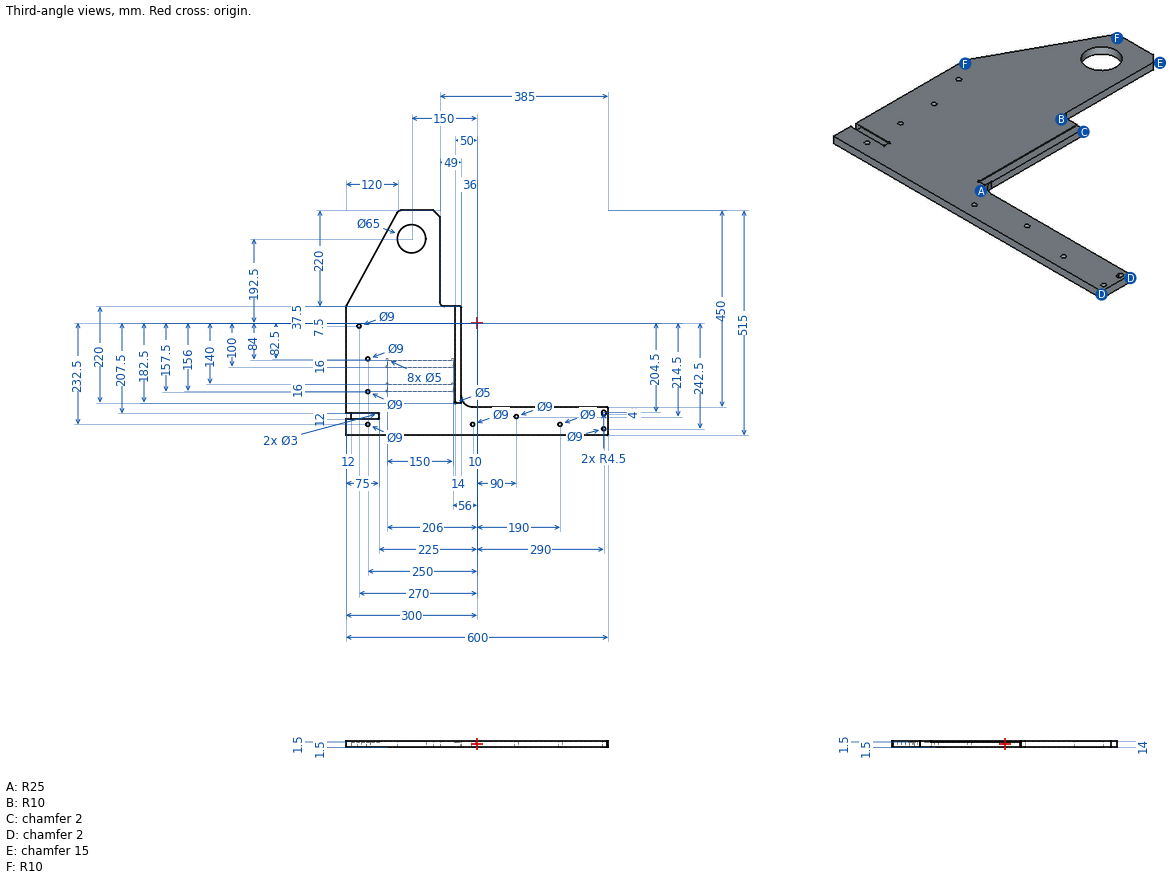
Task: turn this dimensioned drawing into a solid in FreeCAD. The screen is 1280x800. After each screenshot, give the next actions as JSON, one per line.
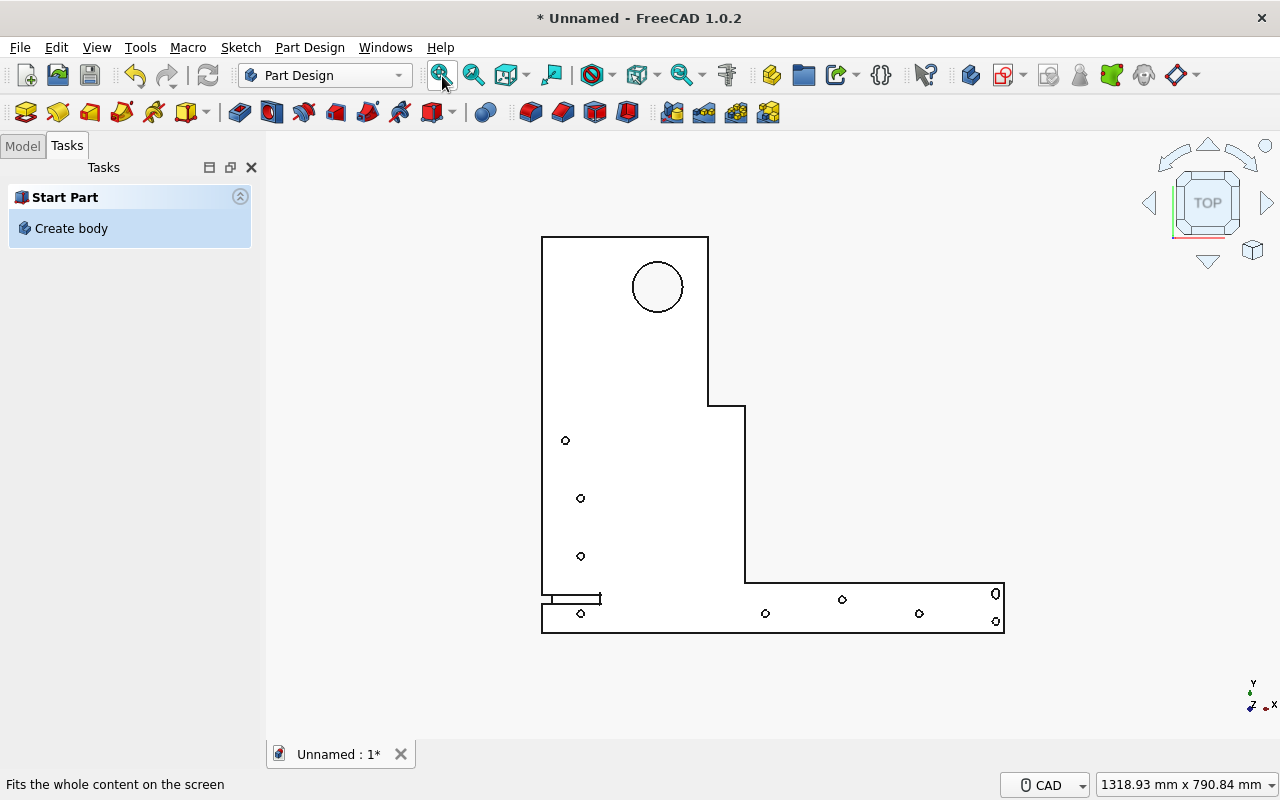
{"action": "key", "text": "1"}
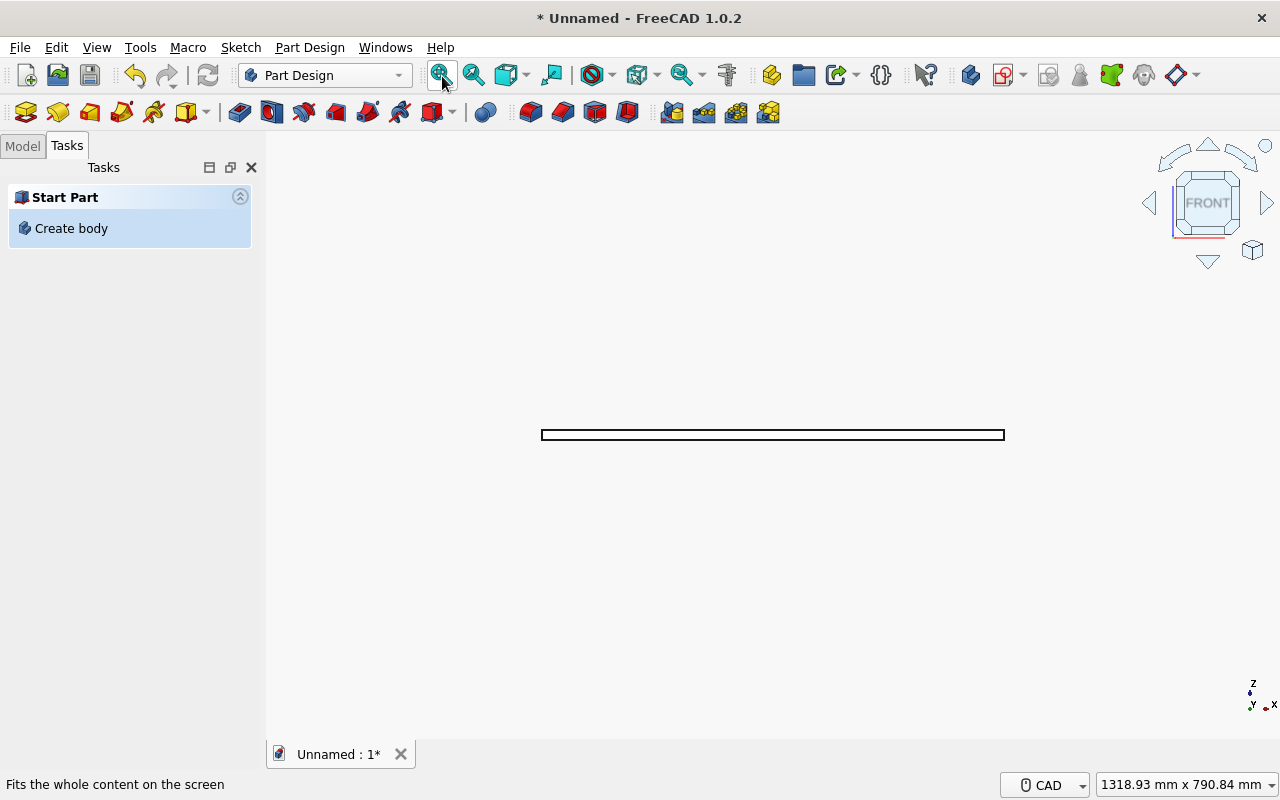
{"action": "scroll", "coordinate": [745, 434], "scroll_direction": "up", "scroll_amount": 7}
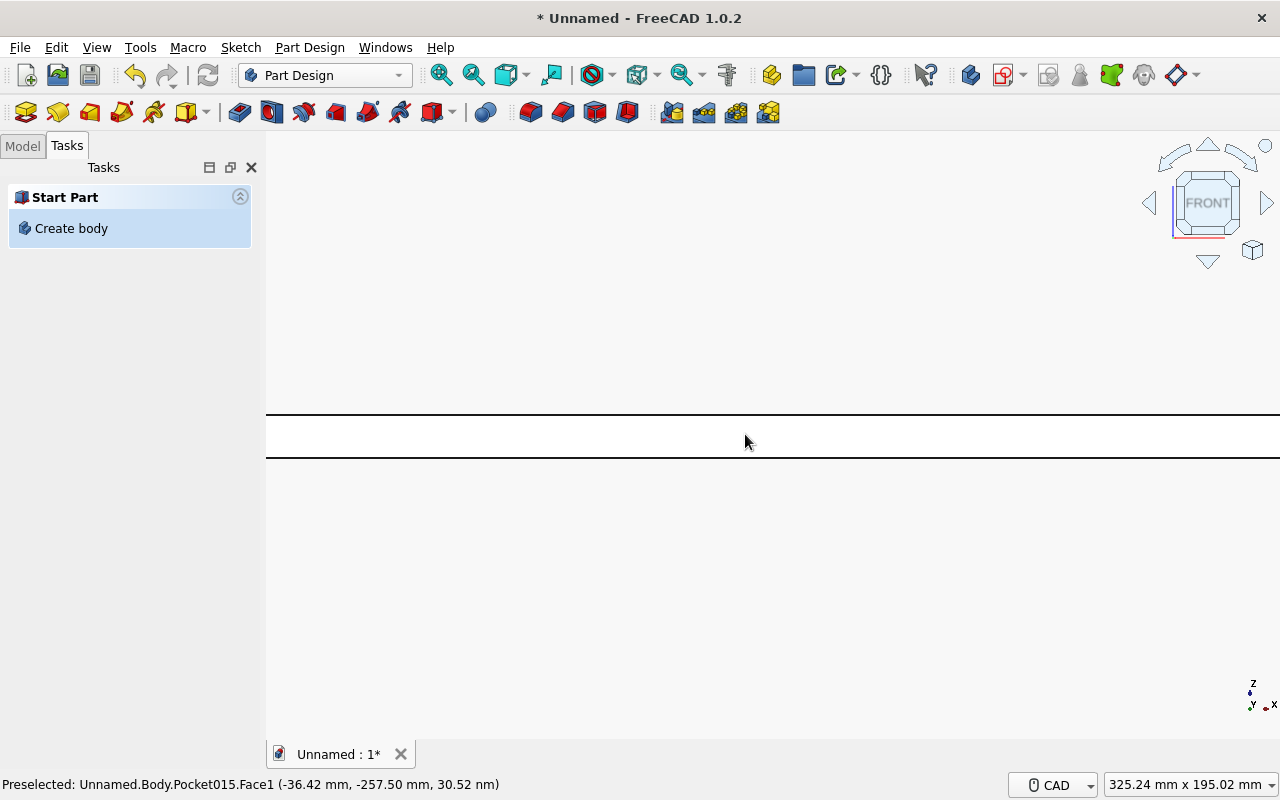
{"action": "left_click", "coordinate": [442, 76]}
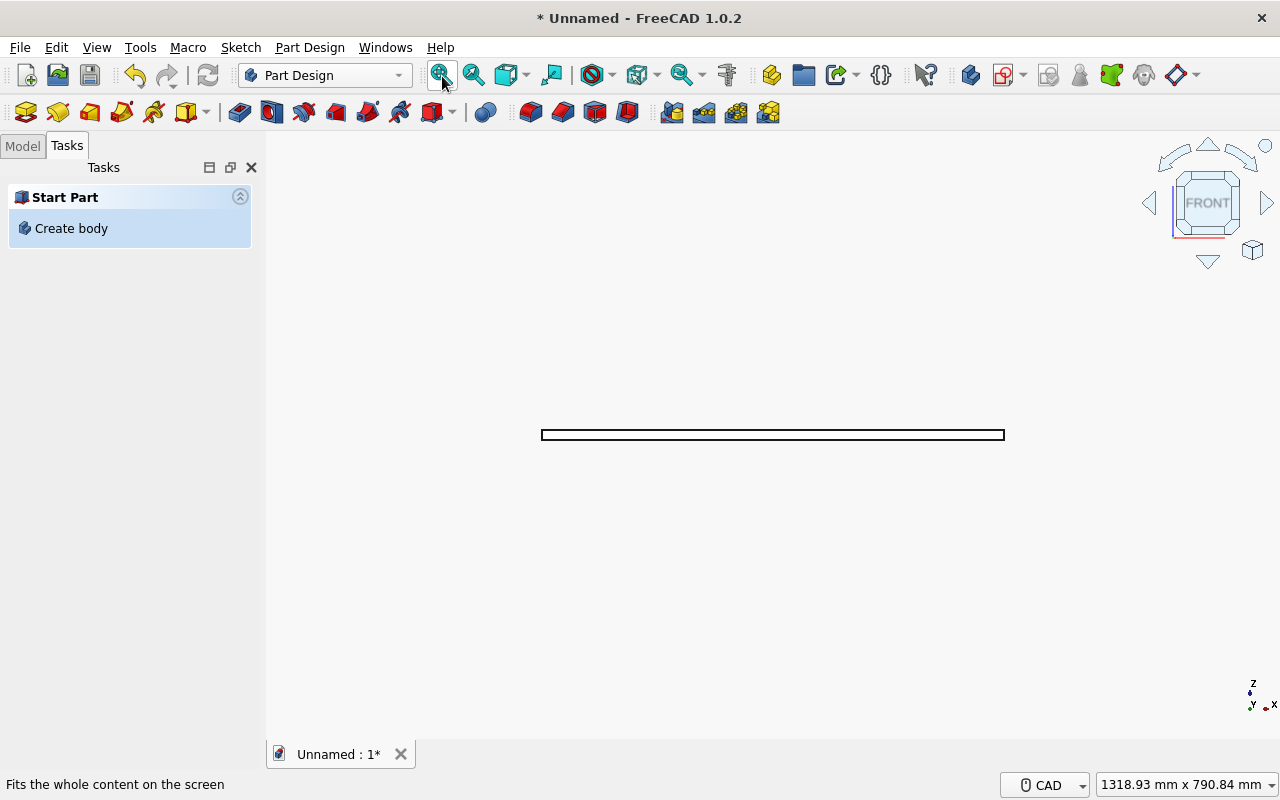
{"action": "key", "text": "3"}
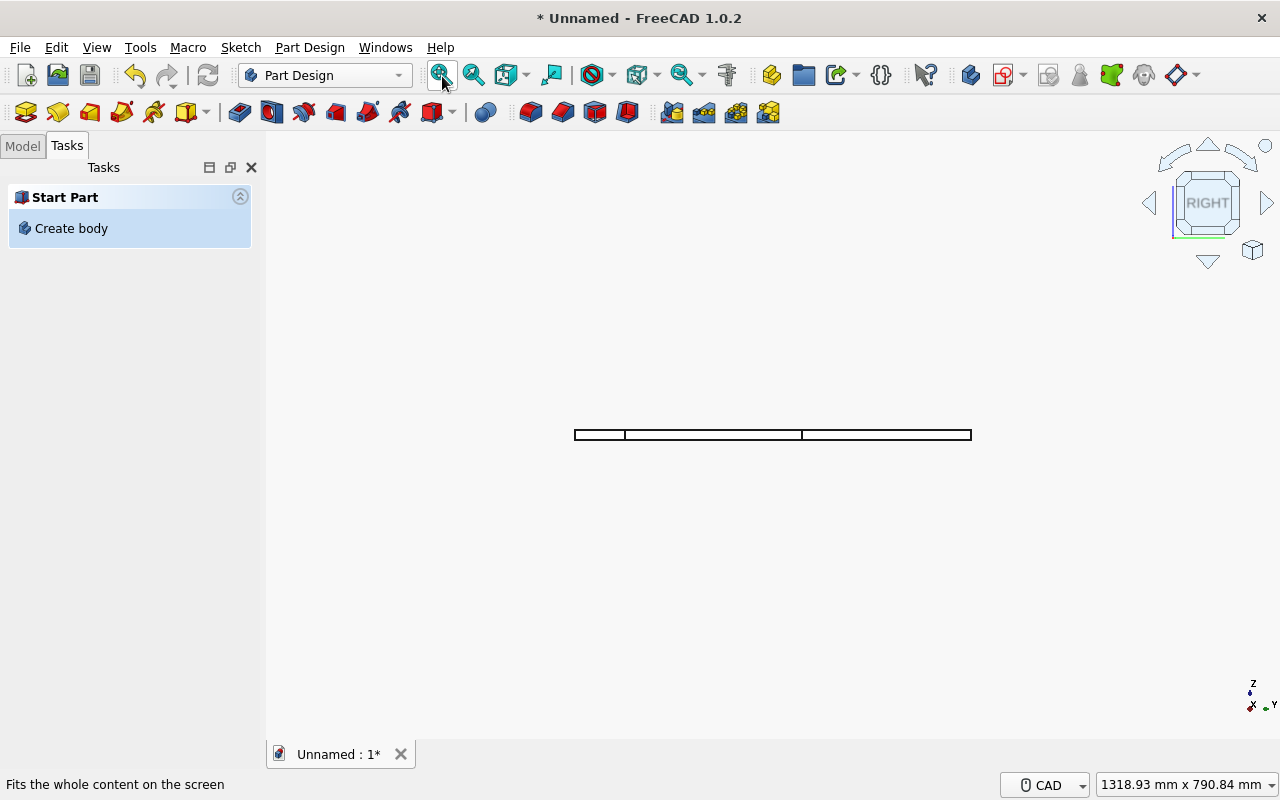
{"action": "left_click", "coordinate": [442, 76]}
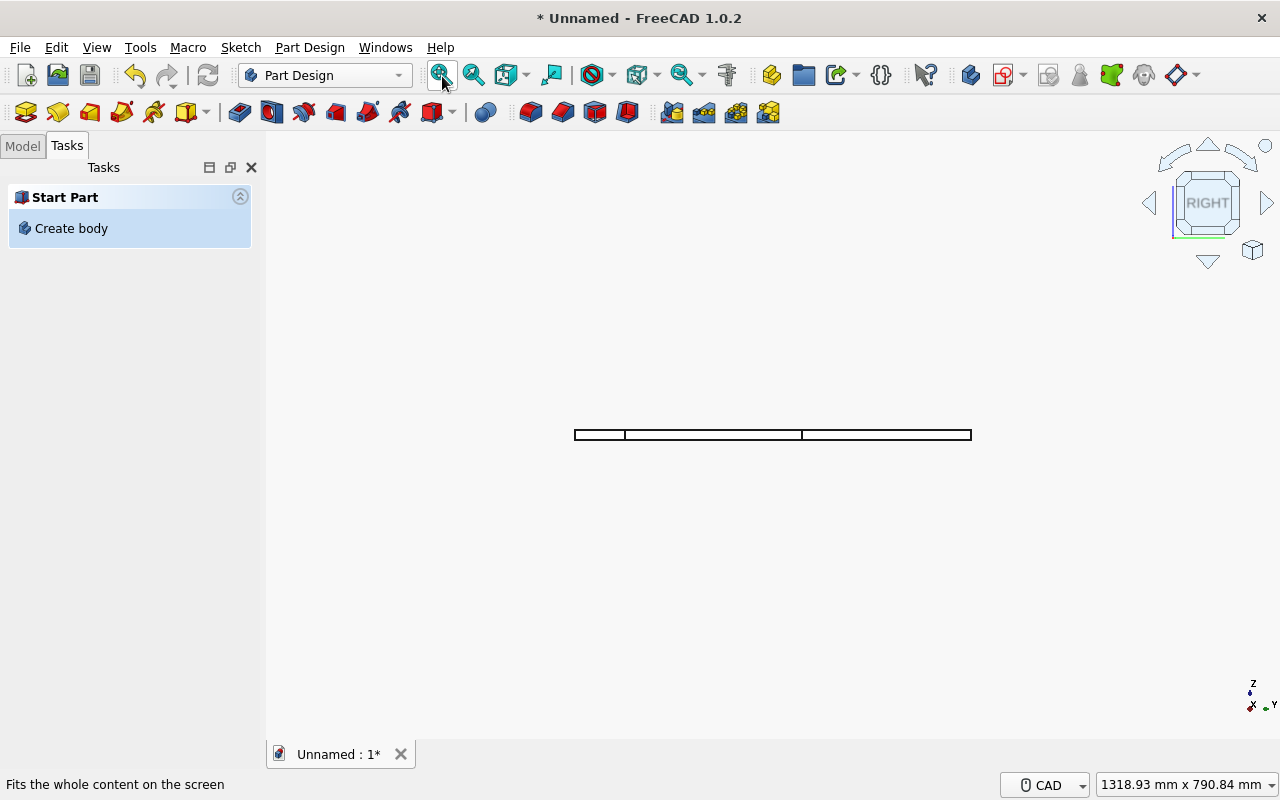
{"action": "scroll", "coordinate": [625, 434], "scroll_direction": "up", "scroll_amount": 7}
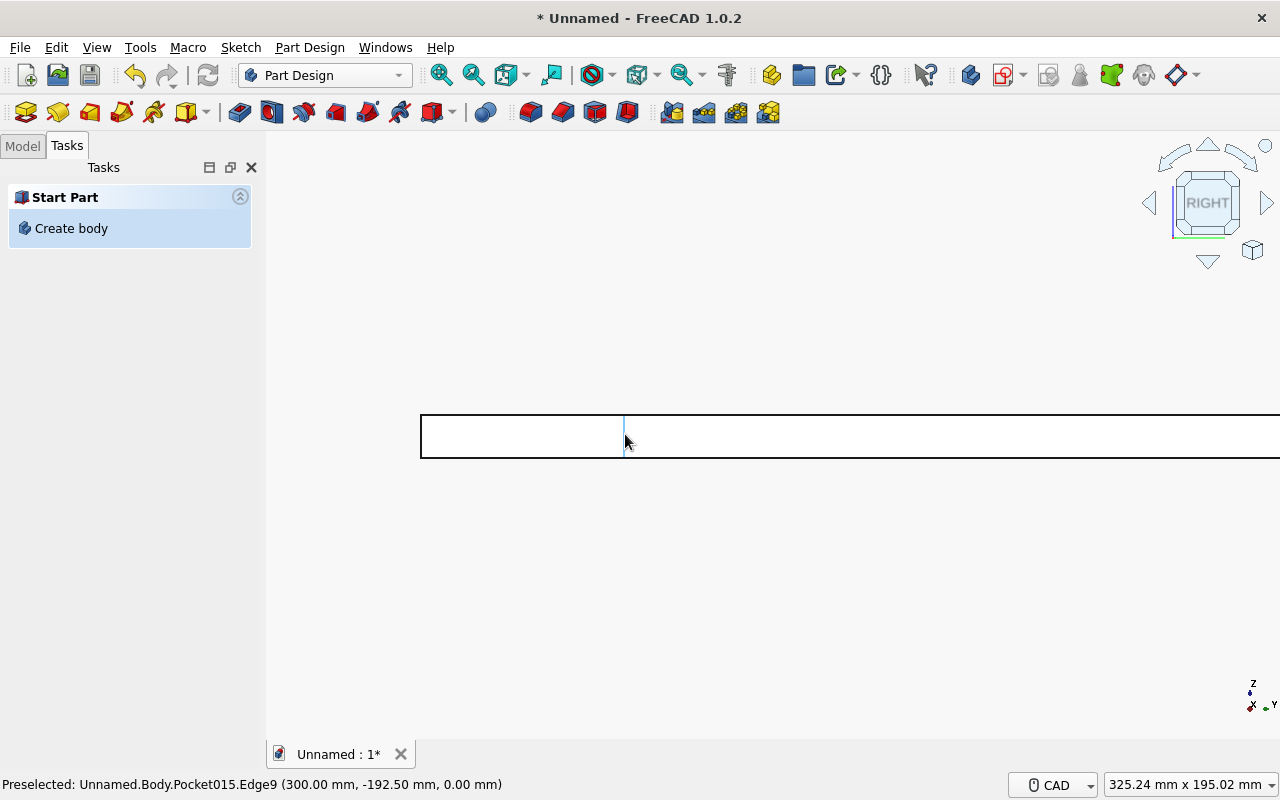
{"action": "left_click", "coordinate": [442, 76]}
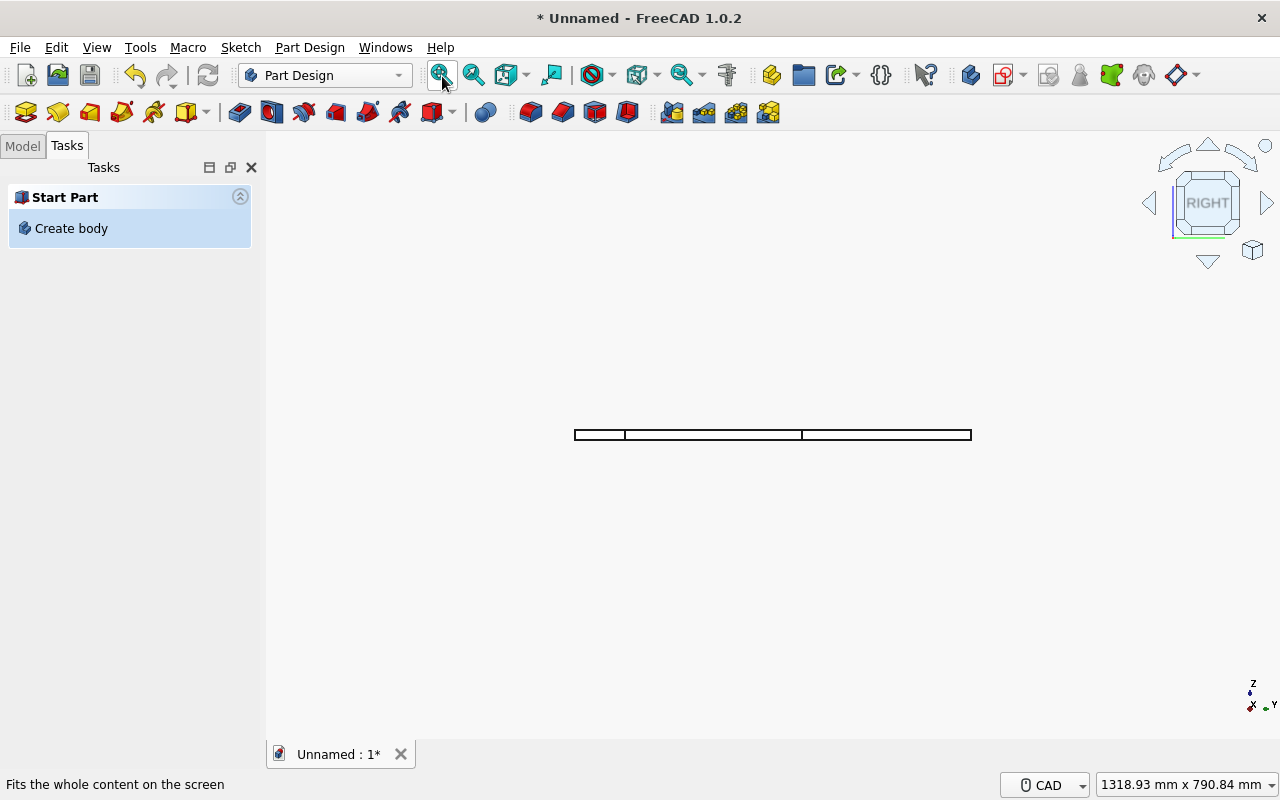
{"action": "key", "text": "5"}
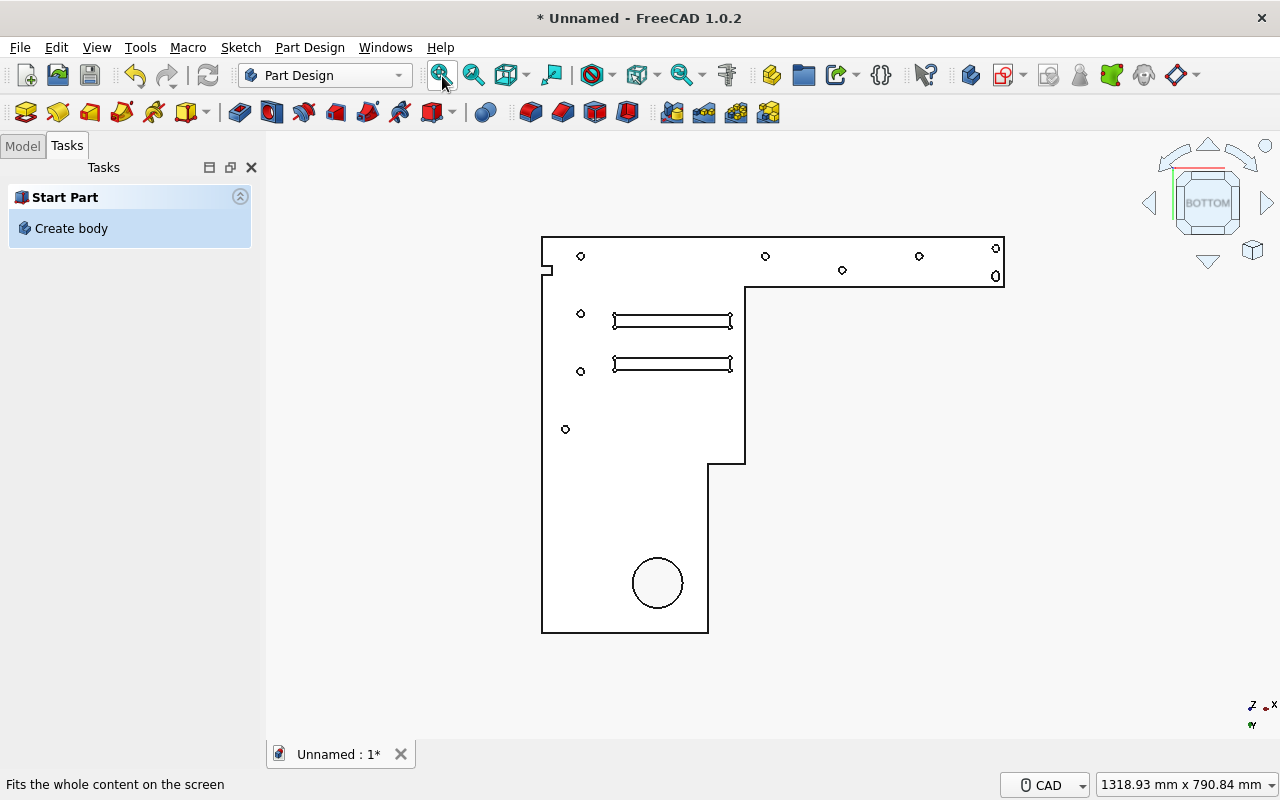
{"action": "scroll", "coordinate": [745, 286], "scroll_direction": "up", "scroll_amount": 7}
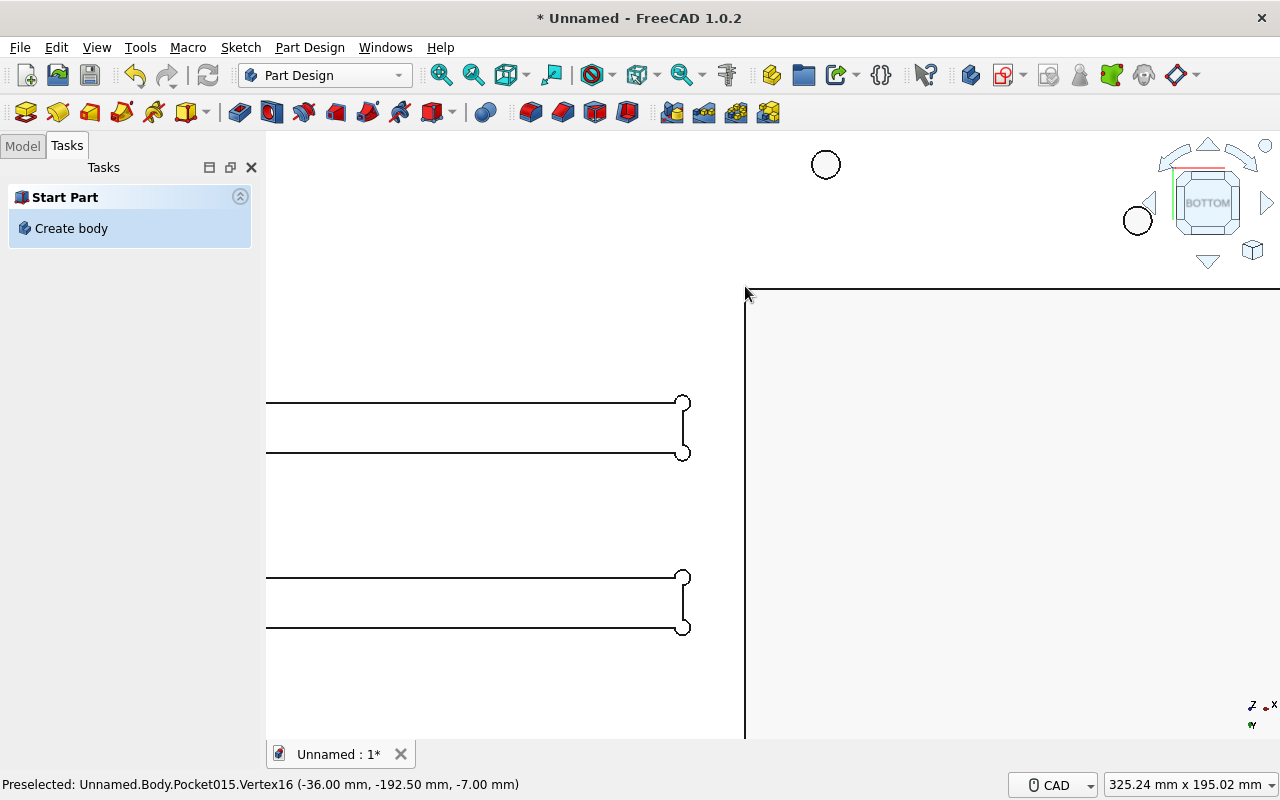
{"action": "left_click", "coordinate": [442, 76]}